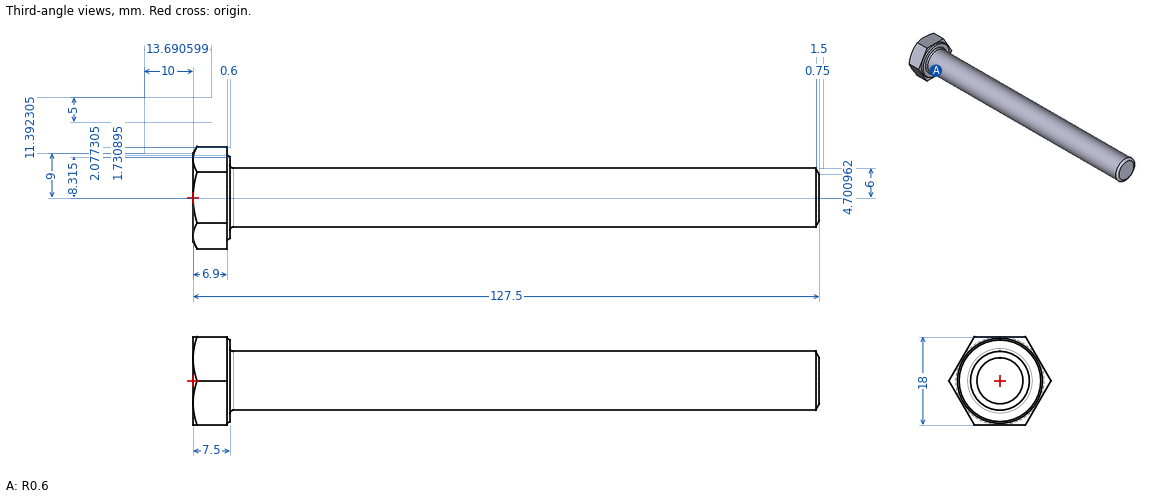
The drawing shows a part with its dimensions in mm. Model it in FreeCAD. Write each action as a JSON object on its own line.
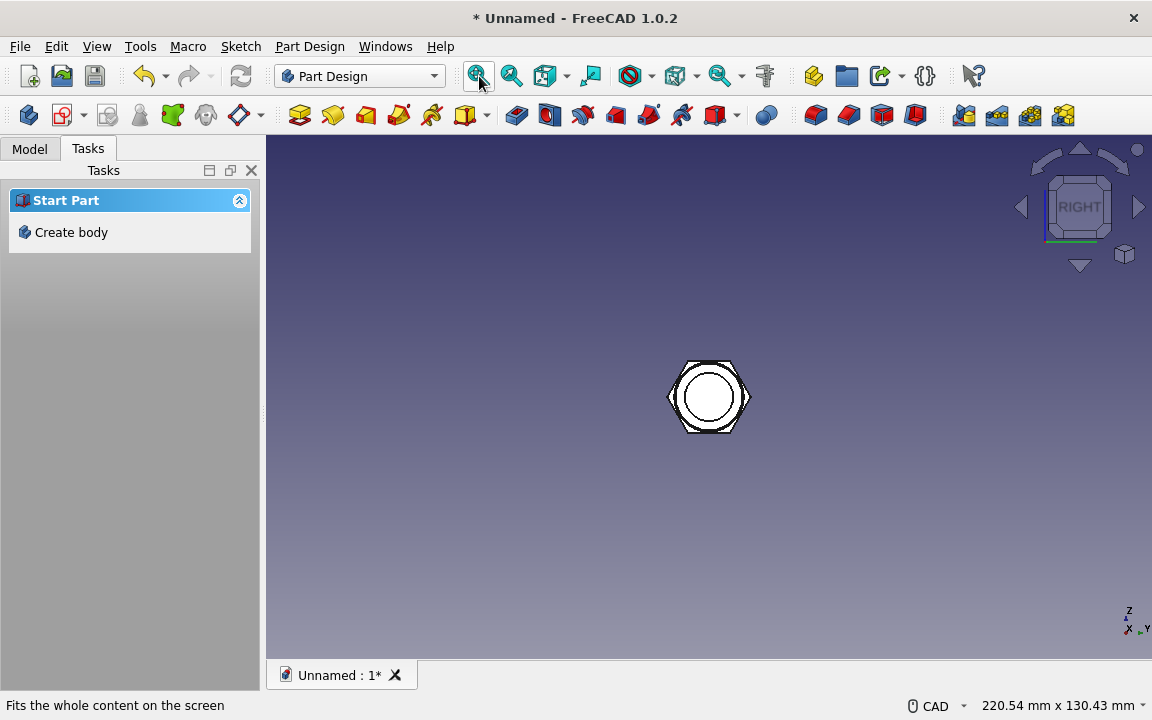
{"action": "key", "text": "5"}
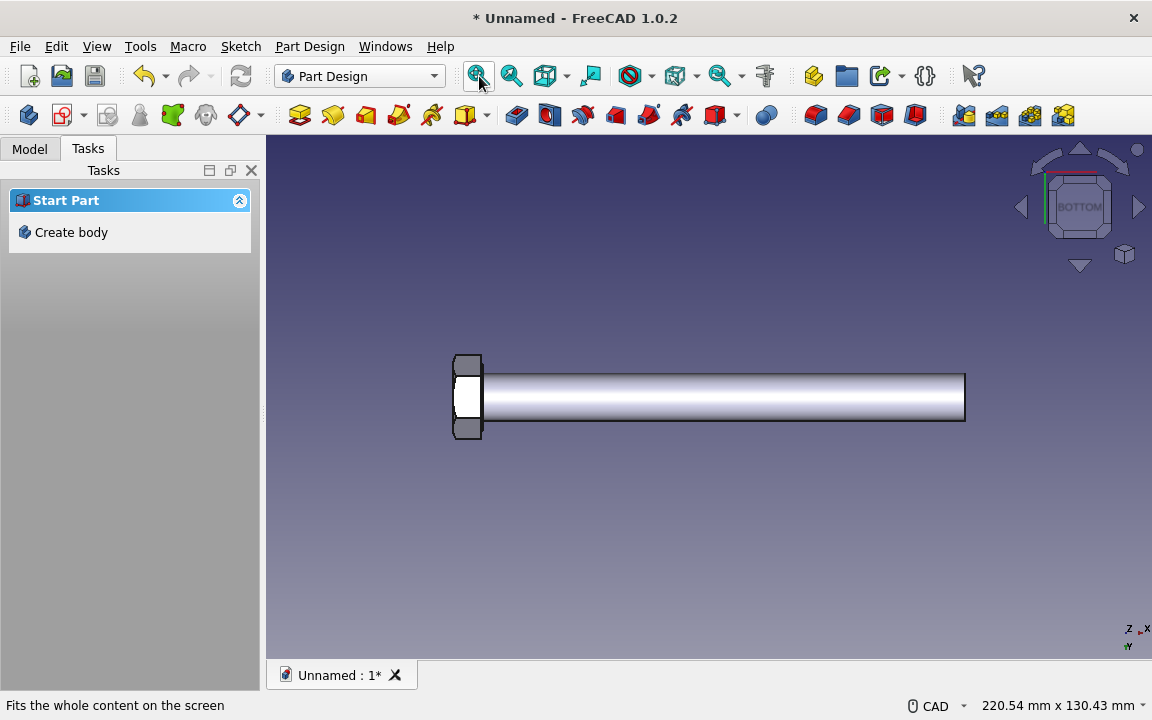
{"action": "key", "text": "4"}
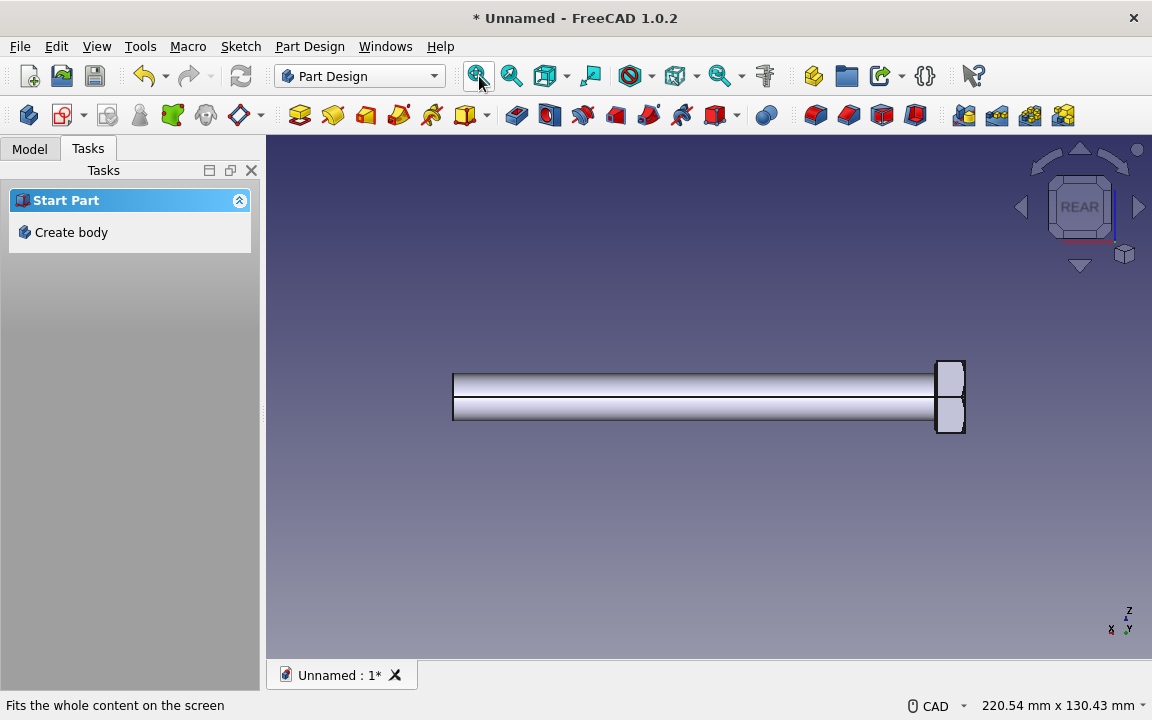
{"action": "key", "text": "6"}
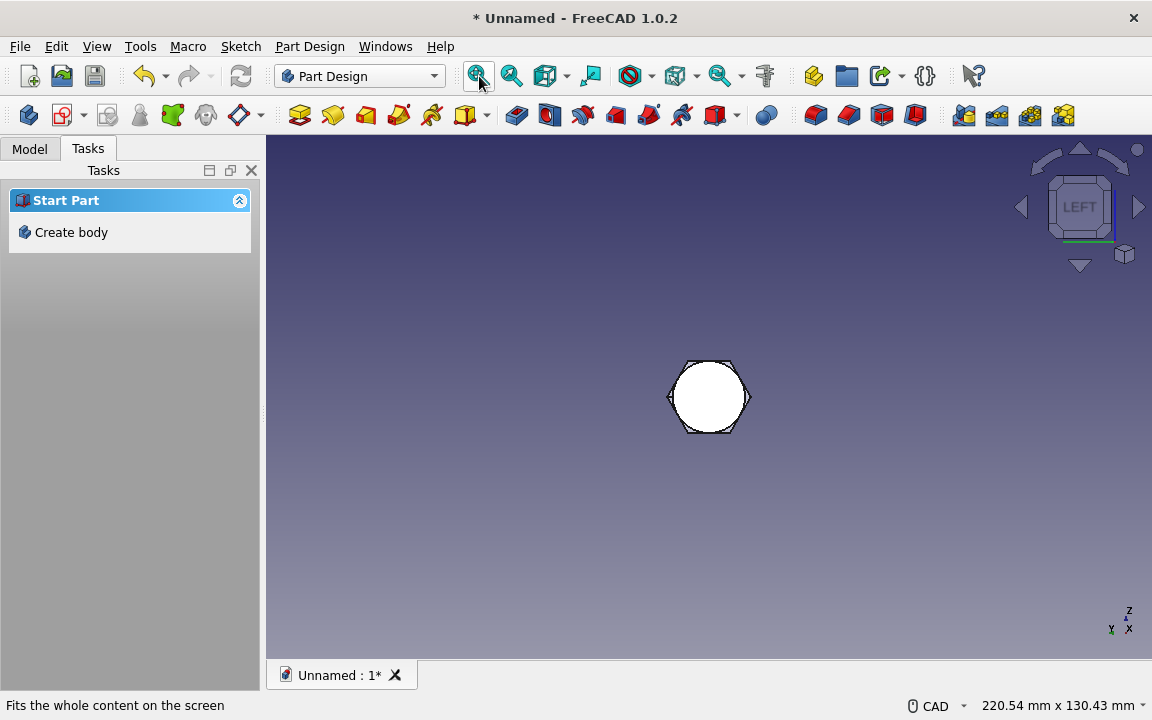
{"action": "left_click", "coordinate": [479, 76]}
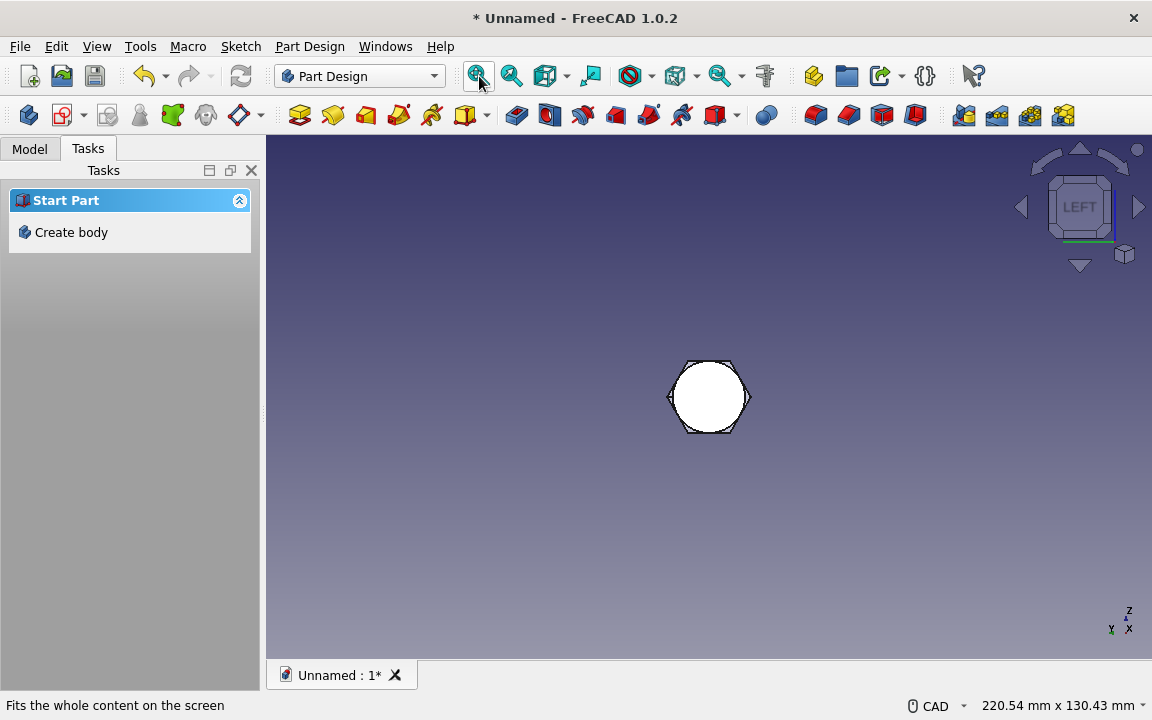
{"action": "key", "text": "v 3"}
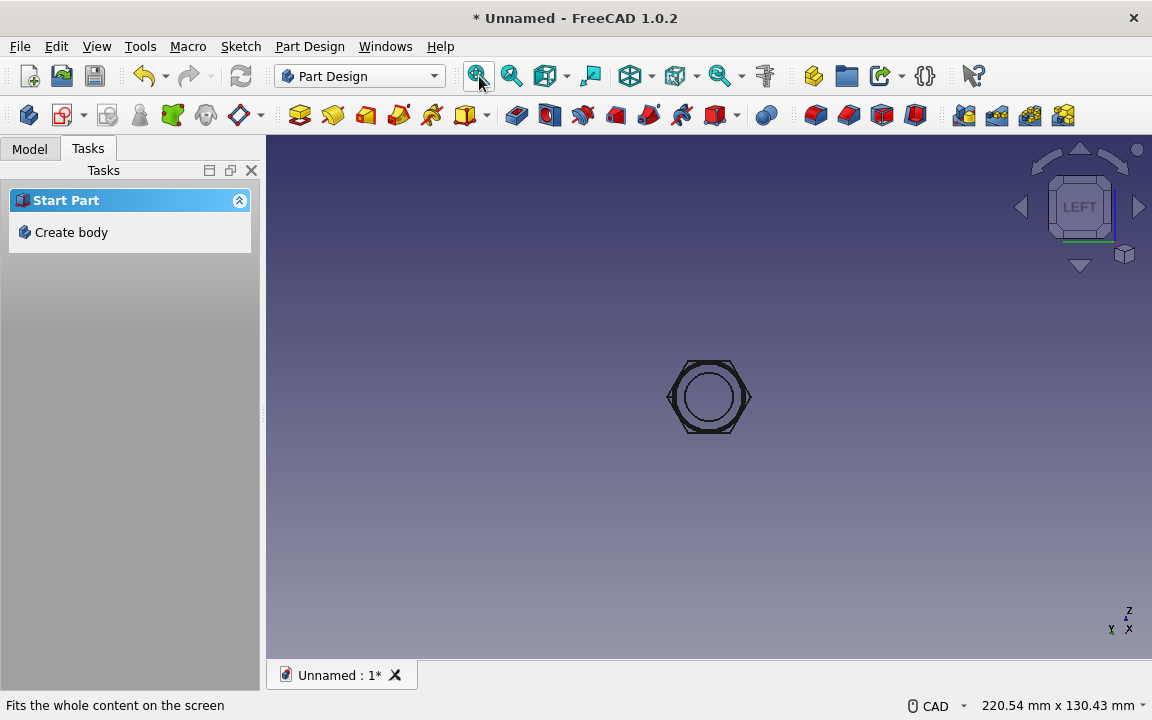
{"action": "key", "text": "0"}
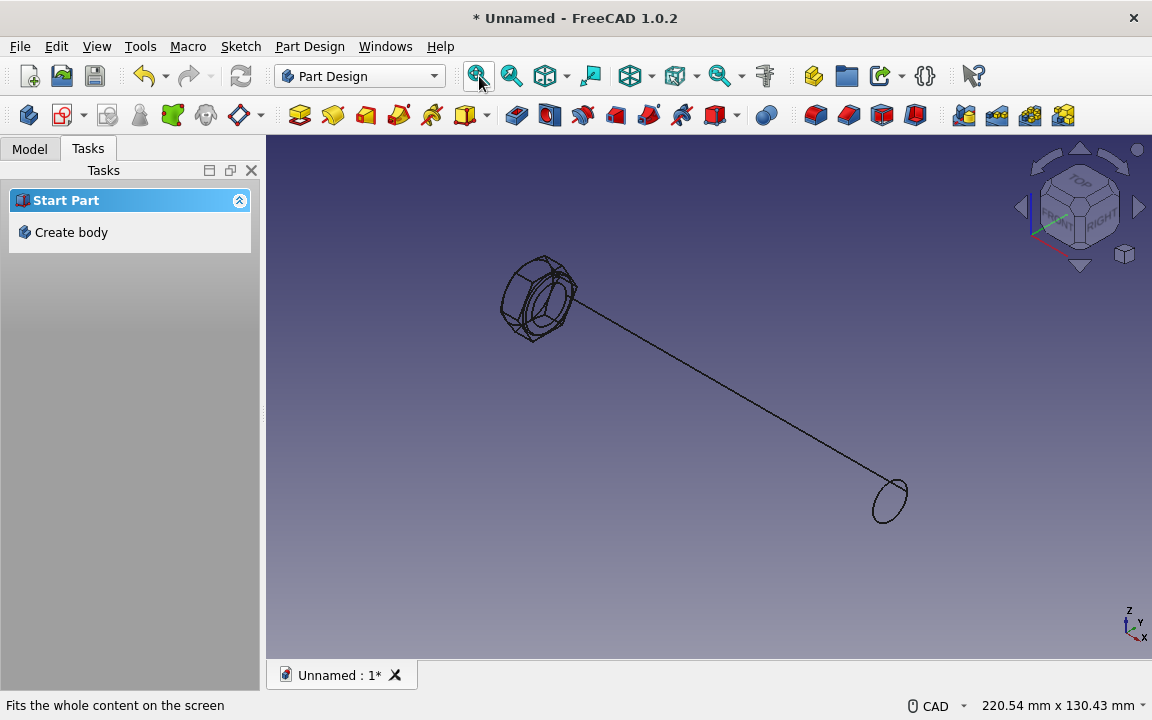
{"action": "left_click", "coordinate": [535, 323]}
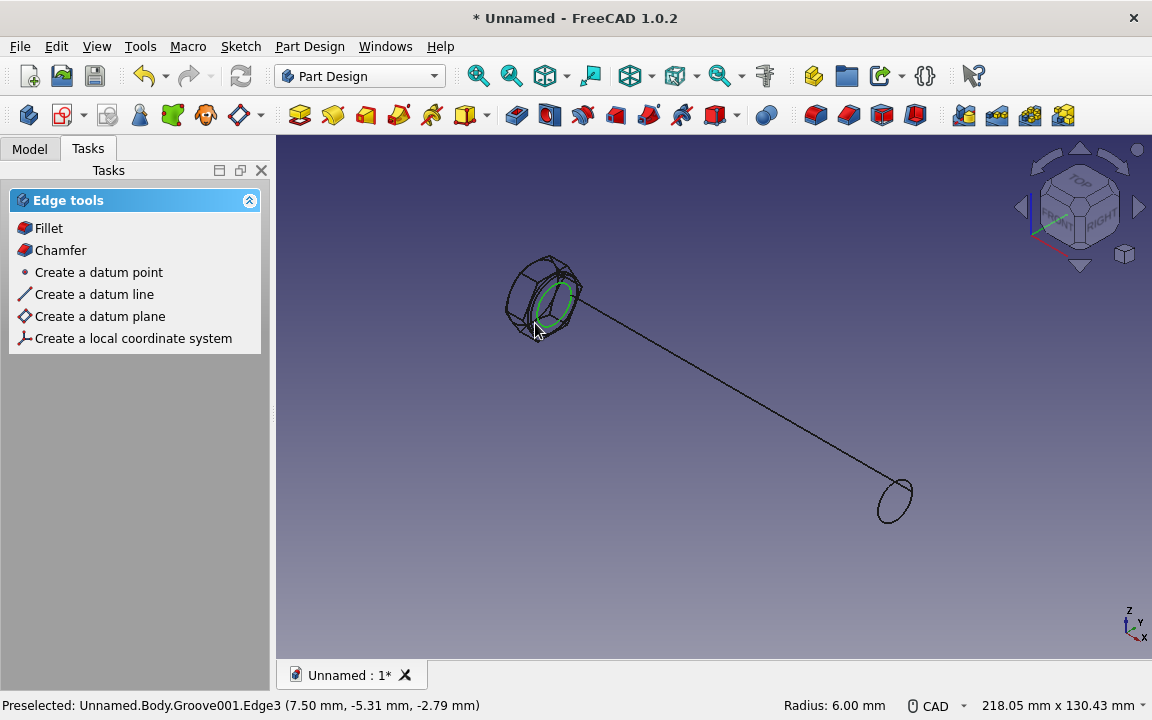
{"action": "key", "text": "v 1"}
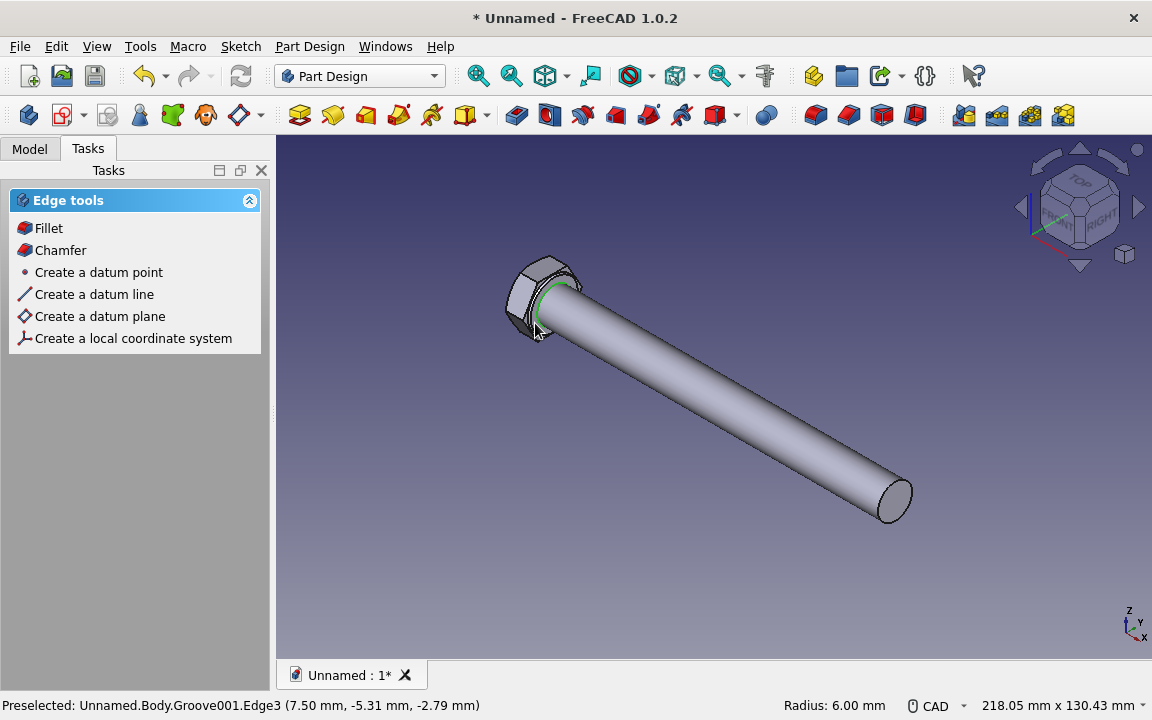
{"action": "left_click", "coordinate": [816, 116]}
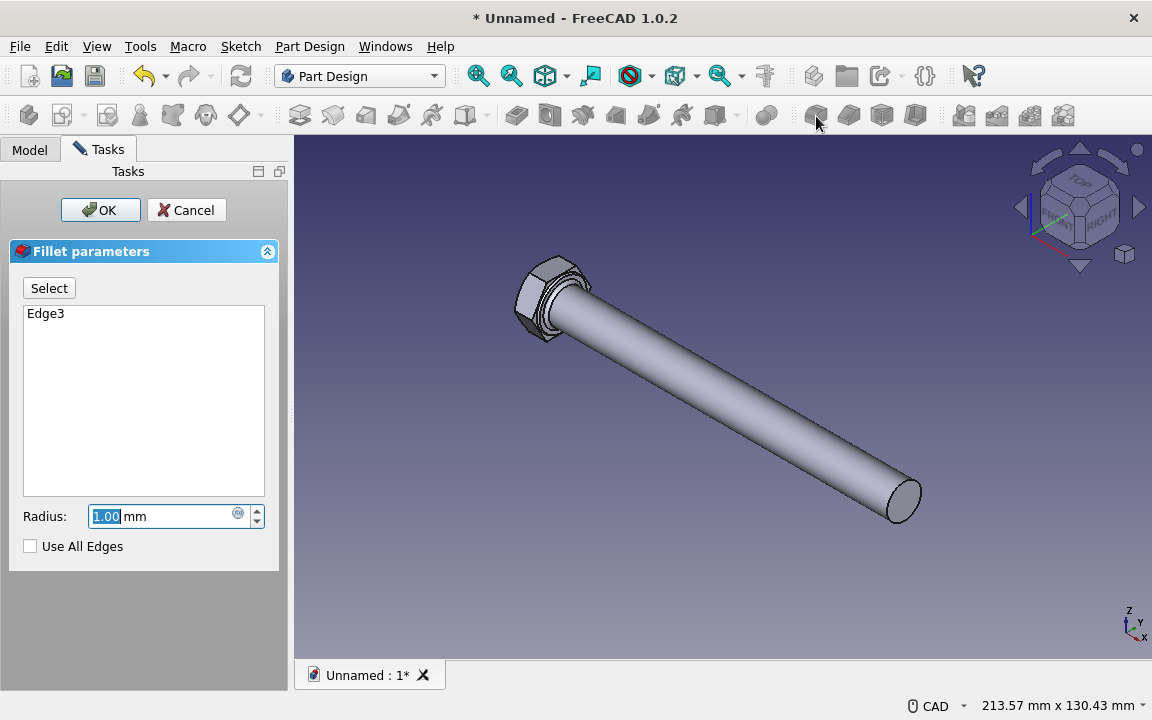
{"action": "type", "text": "0.6"}
{"action": "key", "text": "Tab"}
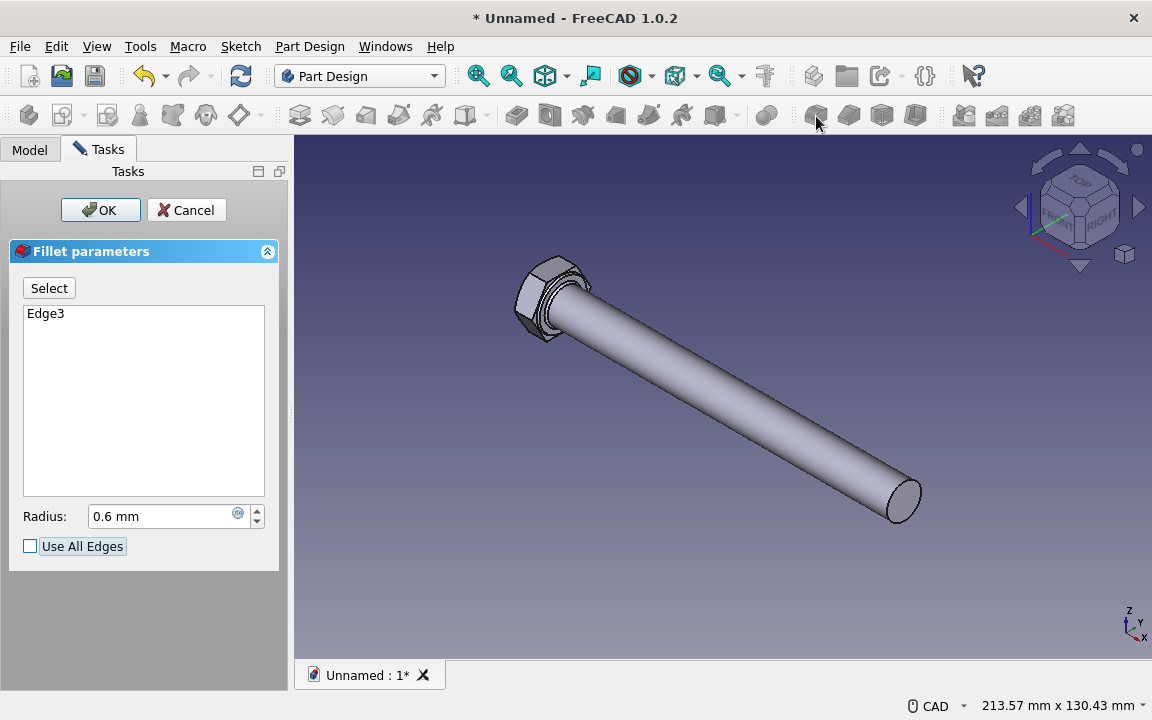
{"action": "left_click", "coordinate": [101, 210]}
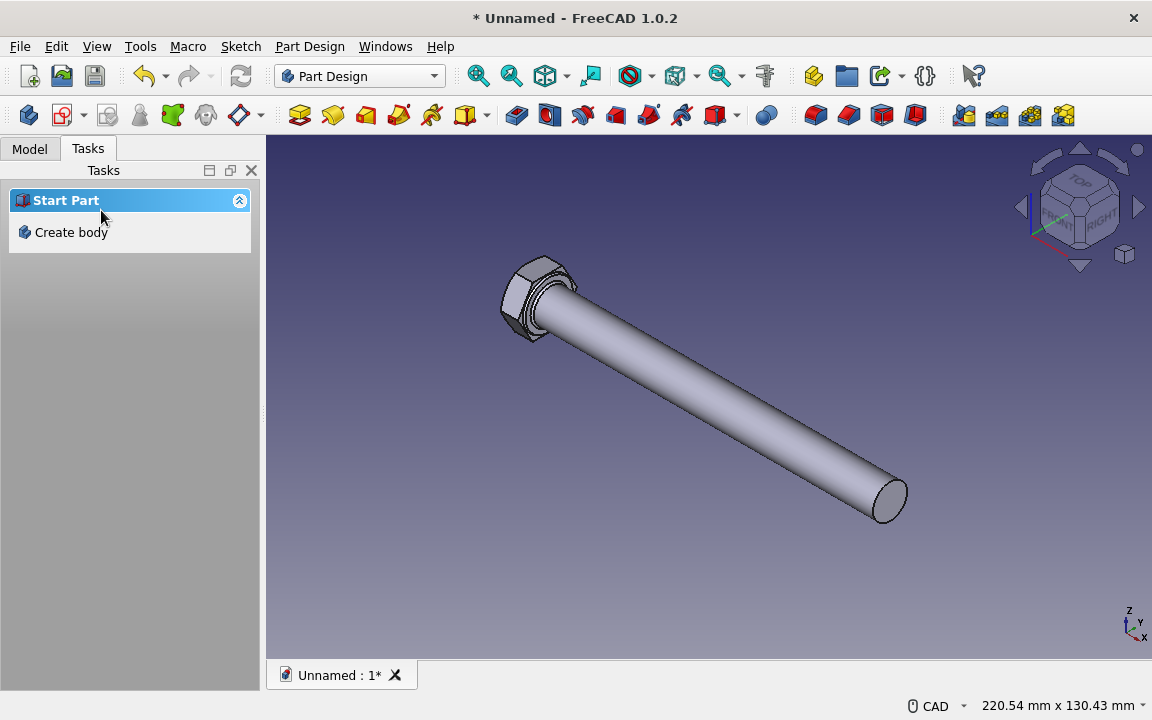
{"action": "left_click", "coordinate": [62, 116]}